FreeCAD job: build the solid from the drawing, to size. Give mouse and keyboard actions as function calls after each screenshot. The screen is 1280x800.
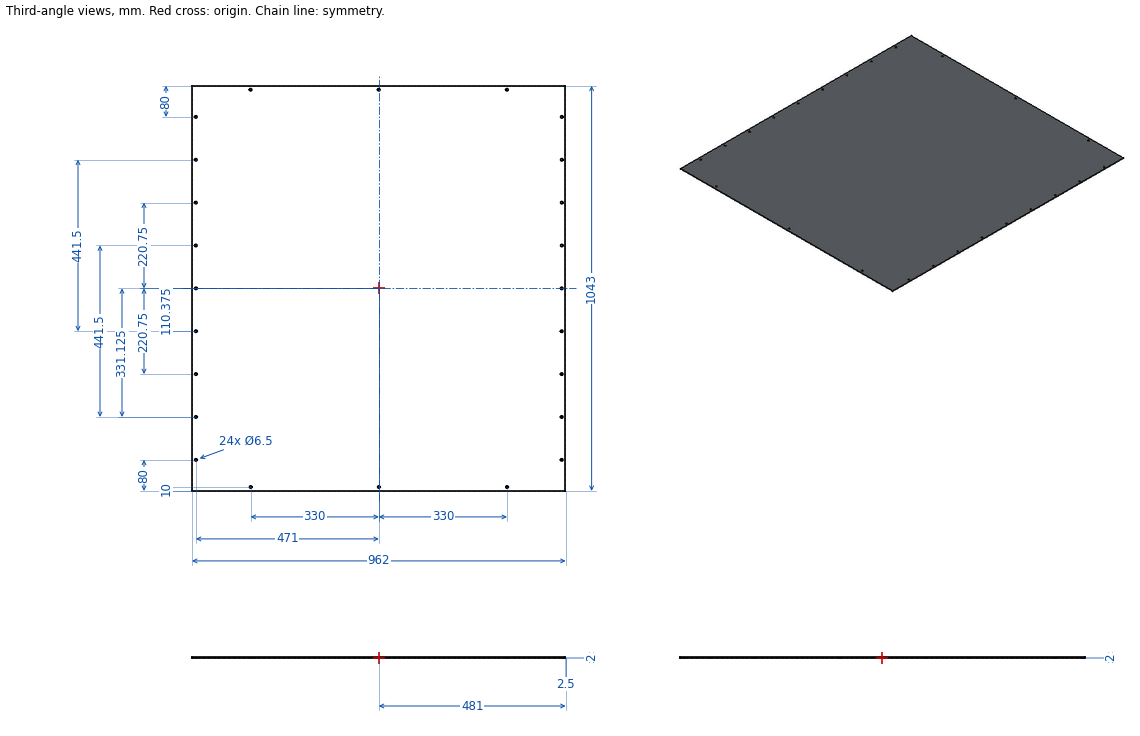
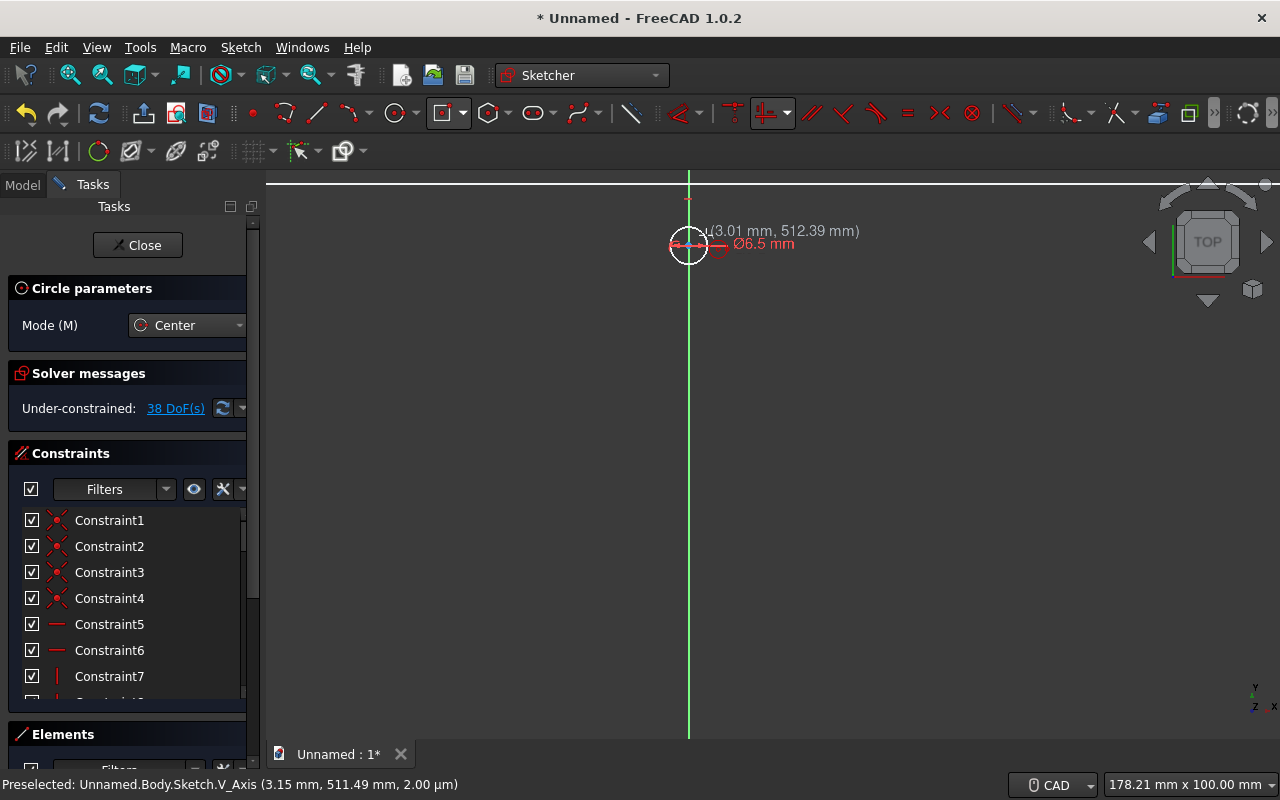
scroll(706, 280, down, 14)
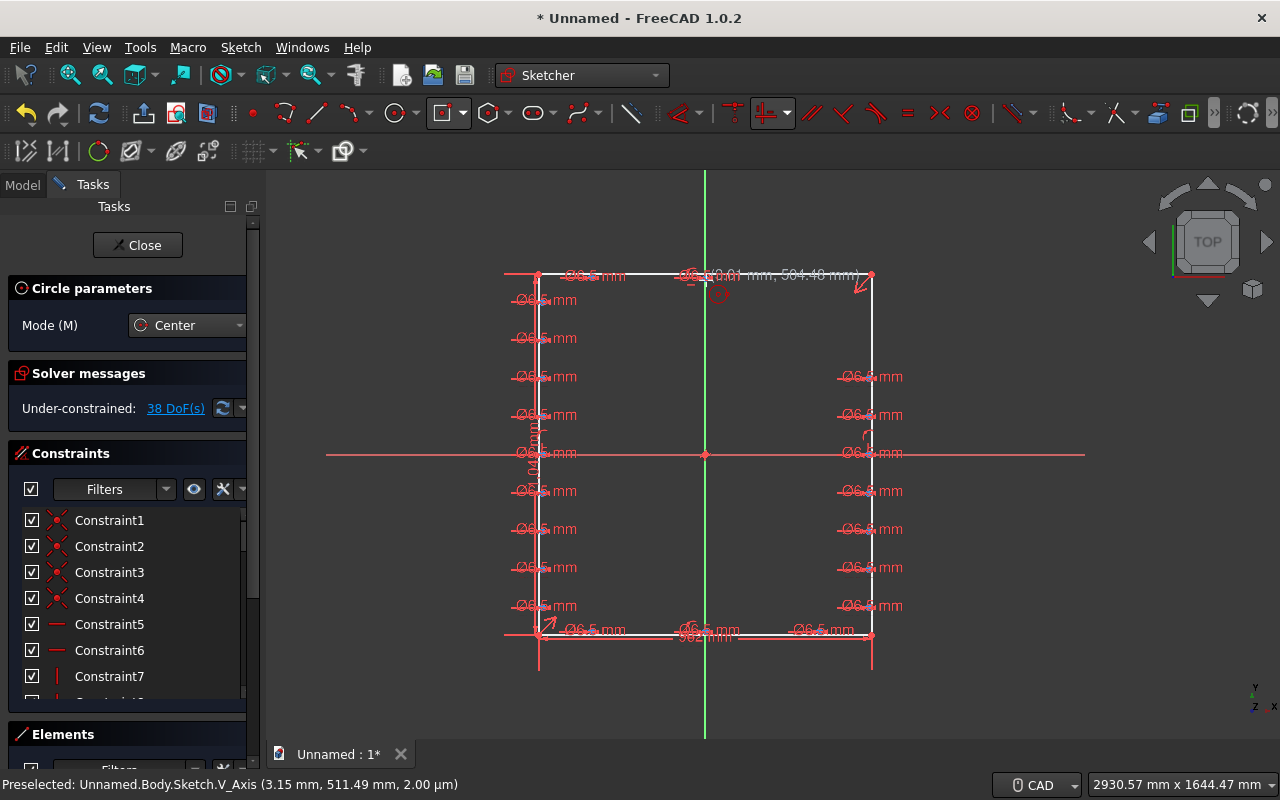
scroll(868, 340, up, 16)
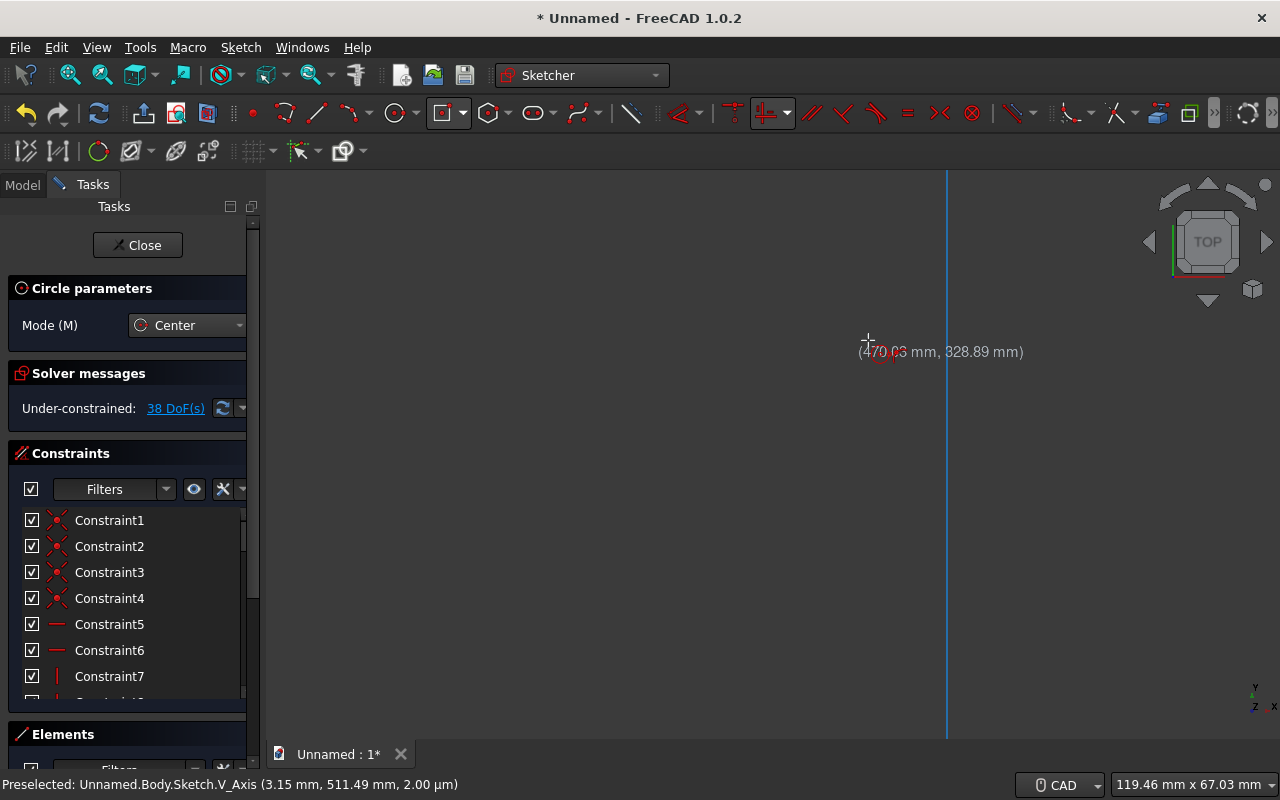
scroll(906, 313, down, 15)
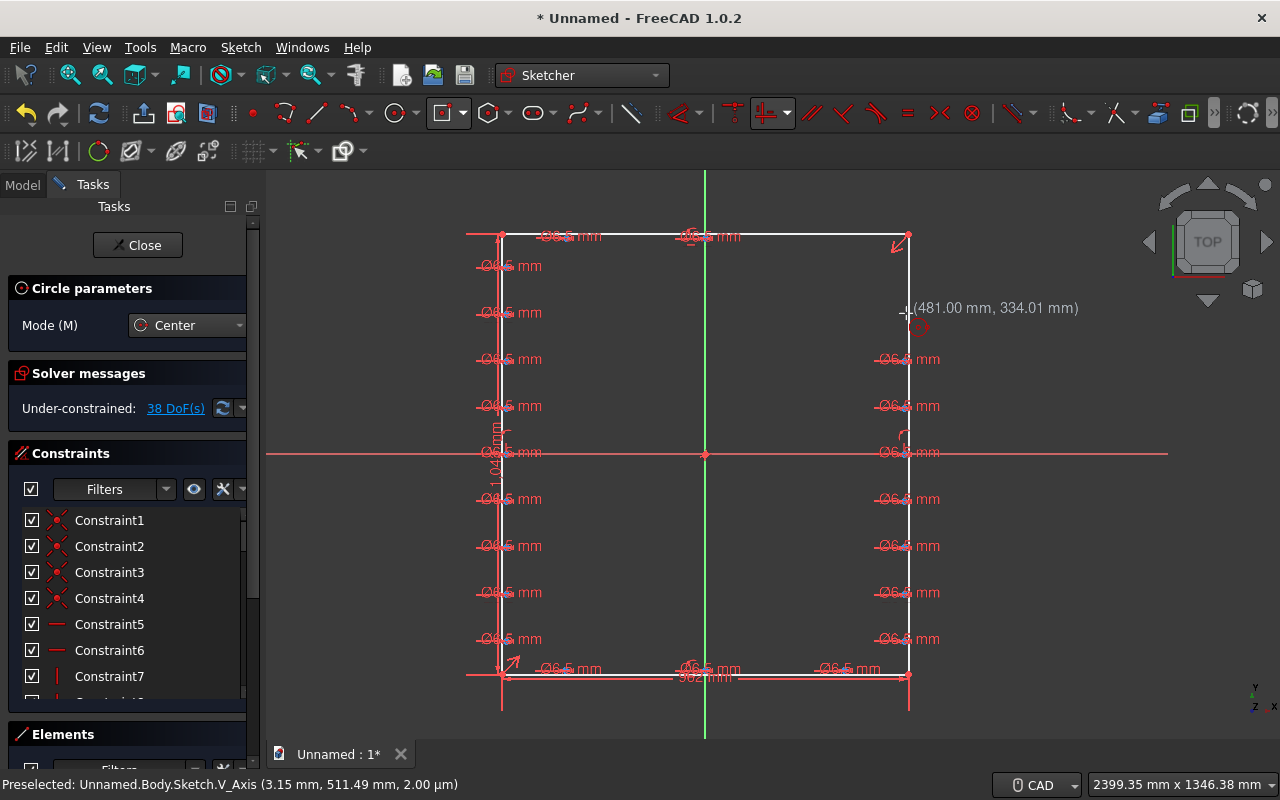
scroll(904, 315, up, 7)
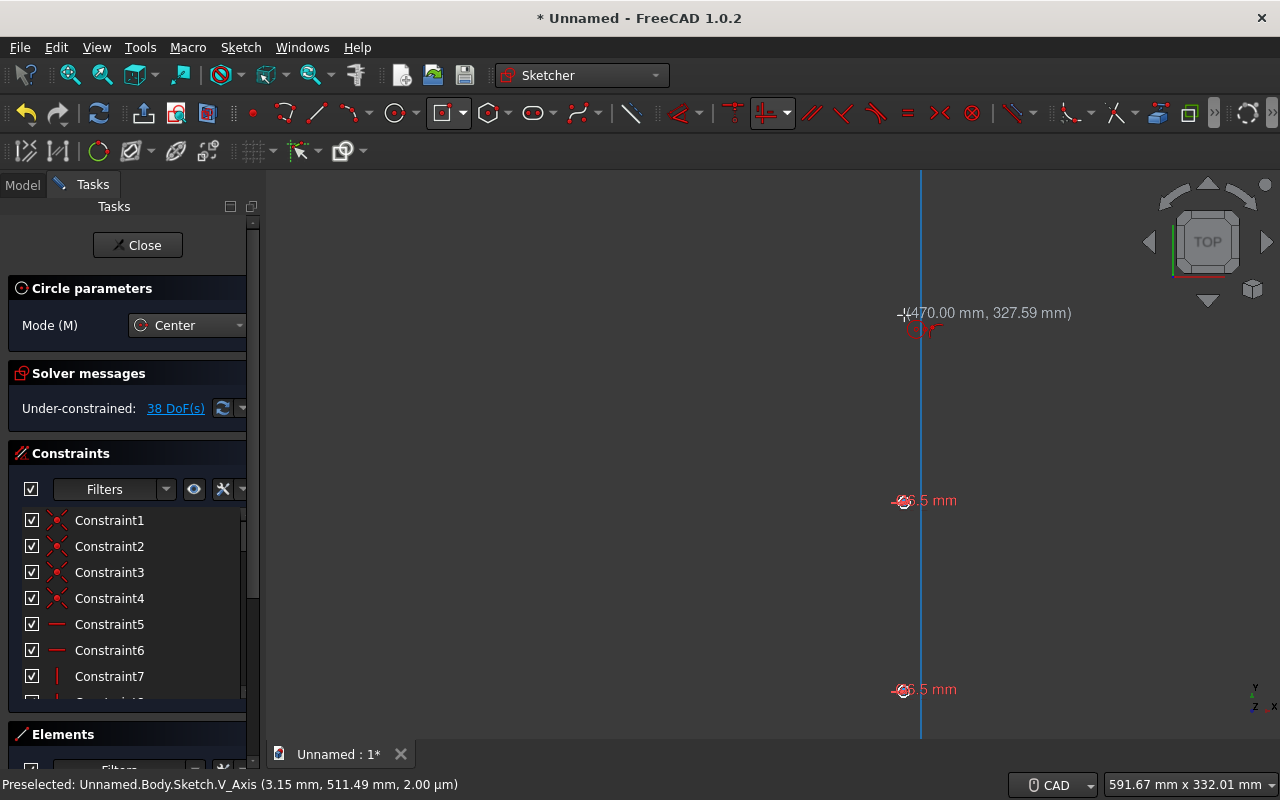
click(904, 312)
move(900, 308)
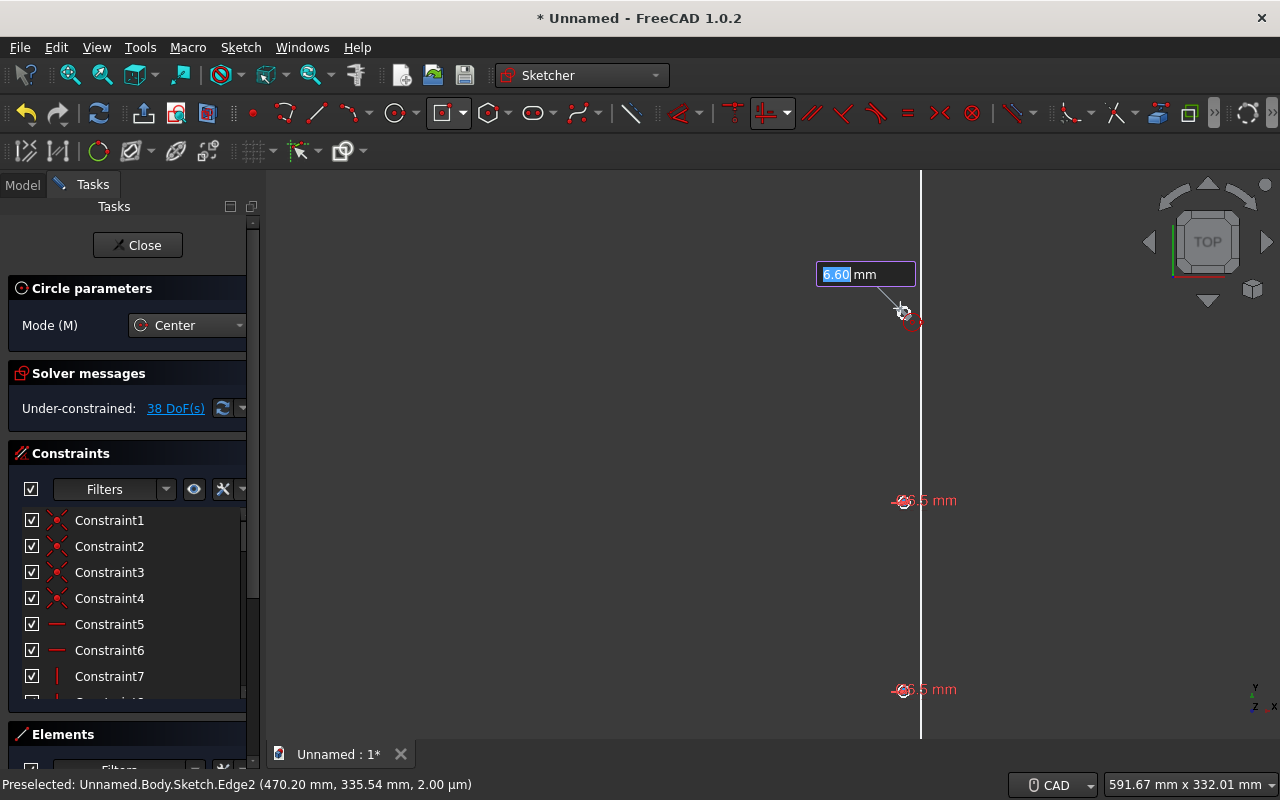
text(6.5)
key(Return)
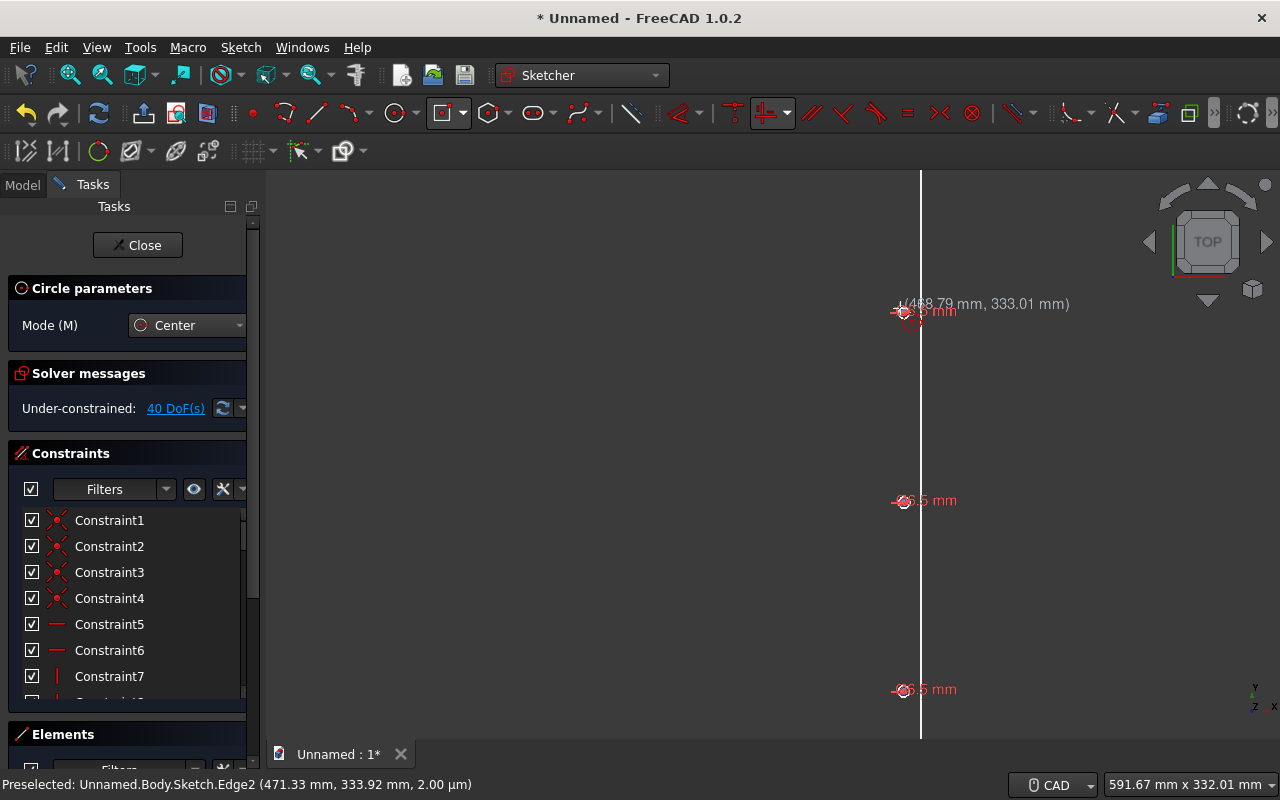
scroll(858, 347, down, 8)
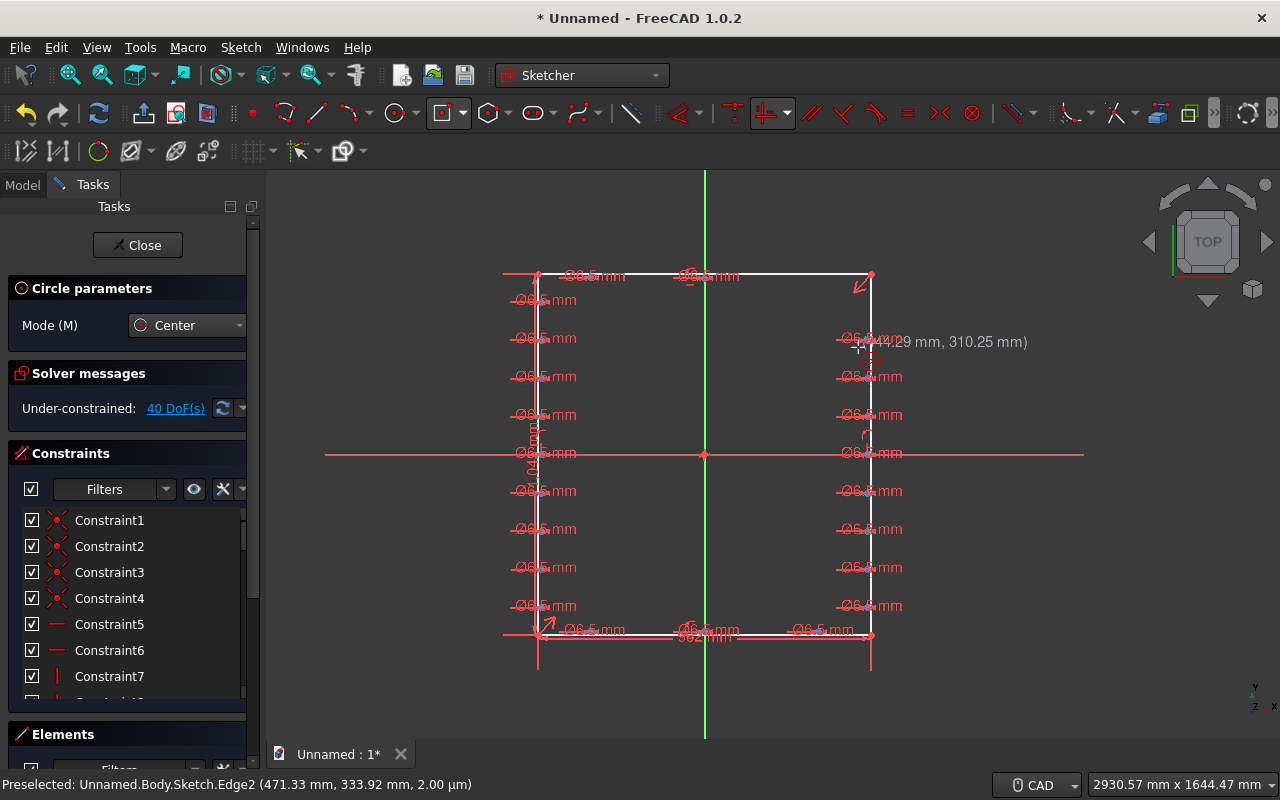
scroll(819, 278, up, 16)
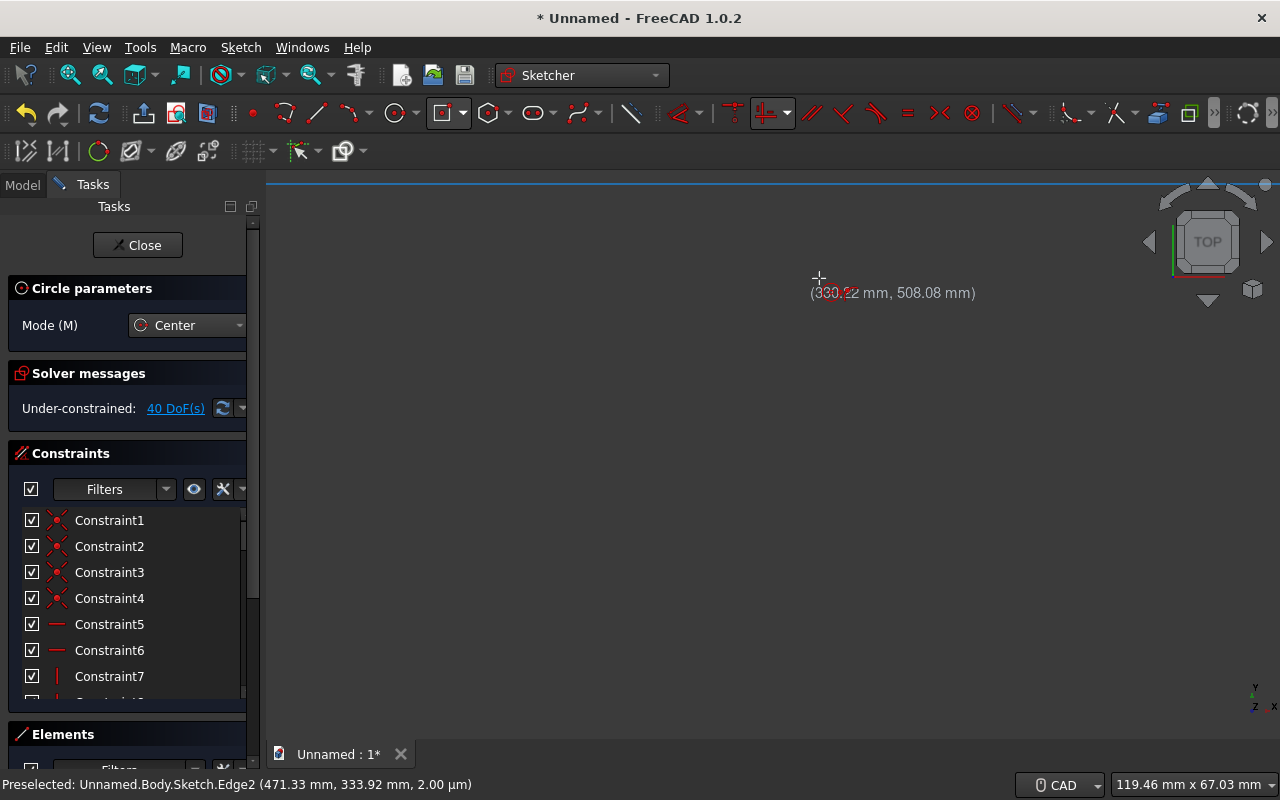
scroll(846, 237, down, 15)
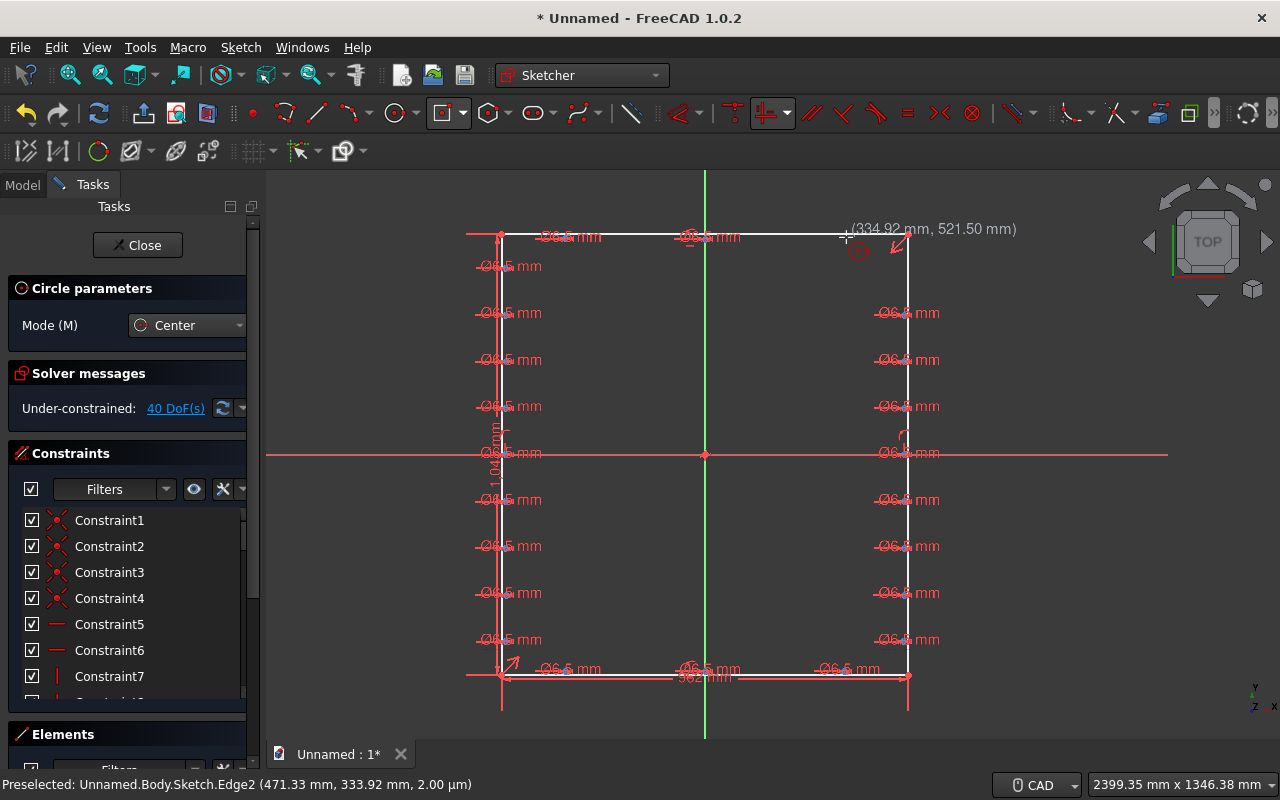
scroll(844, 239, up, 7)